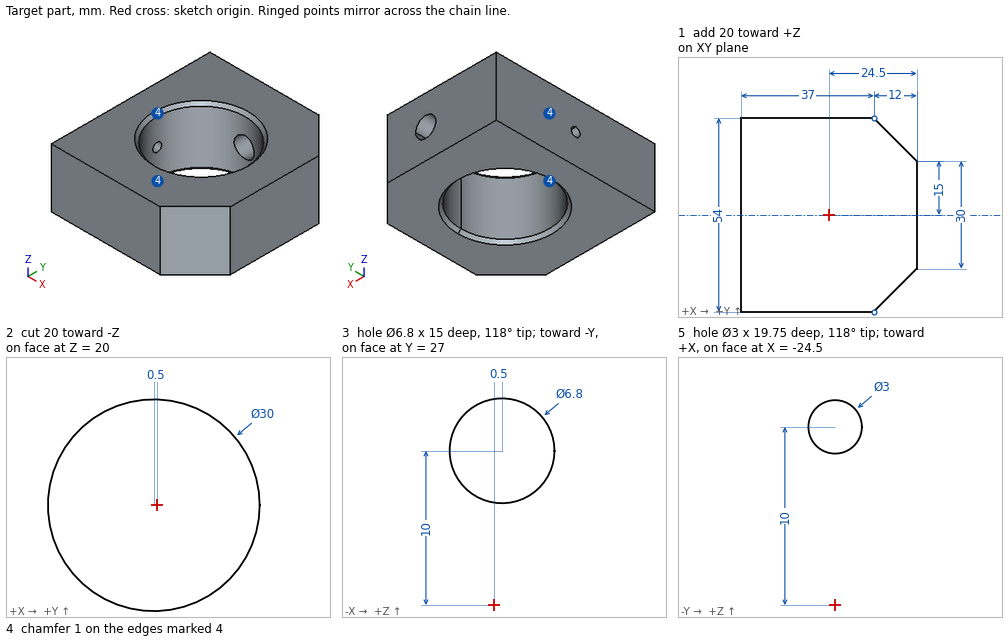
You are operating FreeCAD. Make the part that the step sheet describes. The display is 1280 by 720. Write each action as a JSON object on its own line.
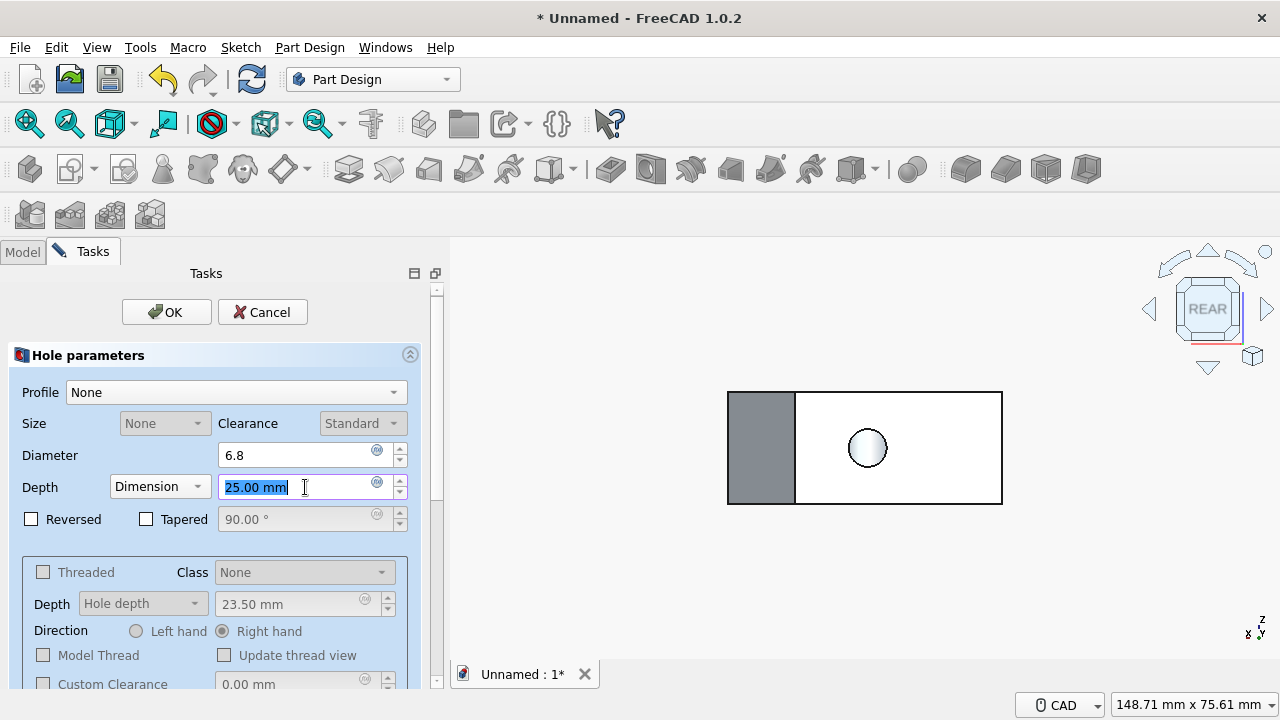
{"action": "type", "text": "15"}
{"action": "key", "text": "Tab"}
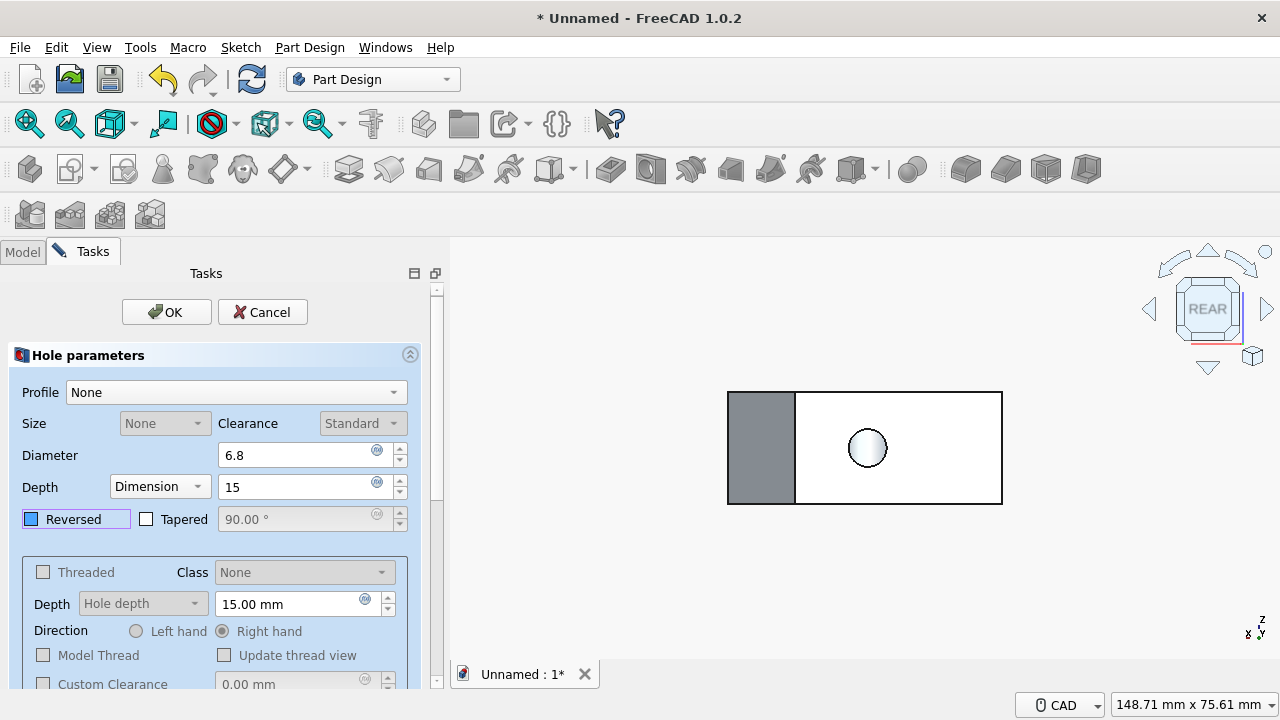
{"action": "left_click", "coordinate": [167, 312]}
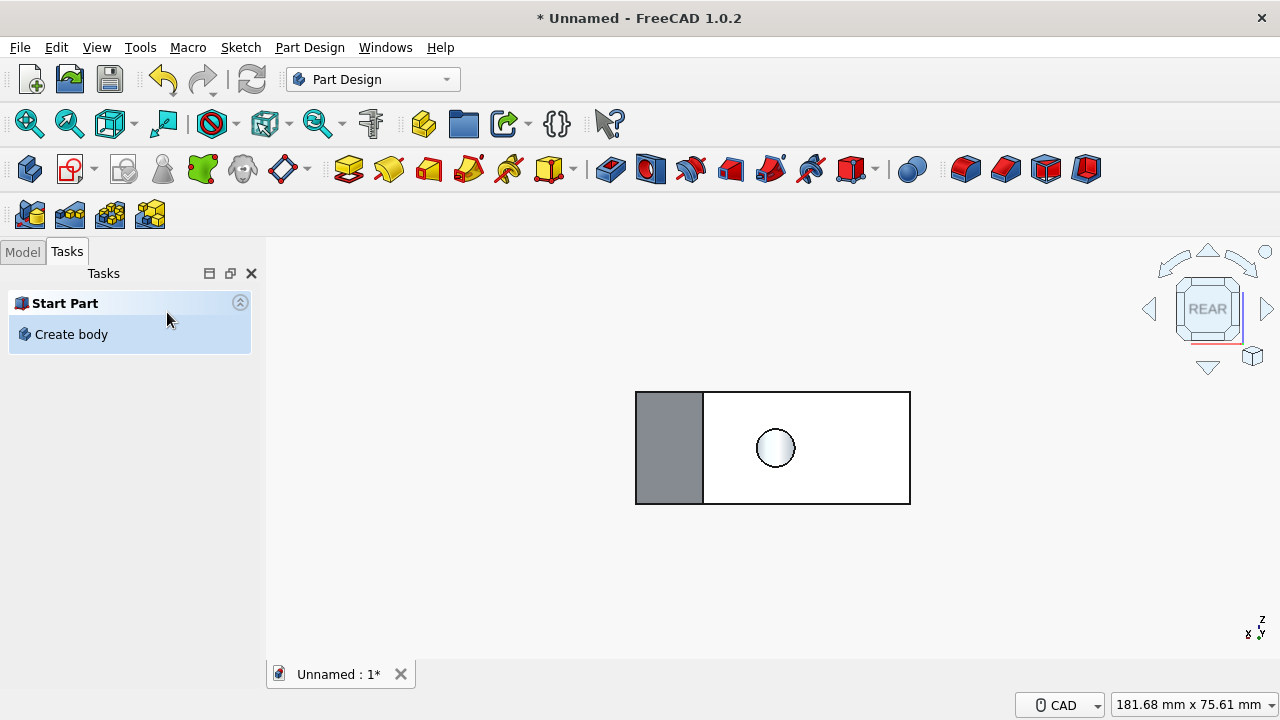
{"action": "left_click", "coordinate": [30, 124]}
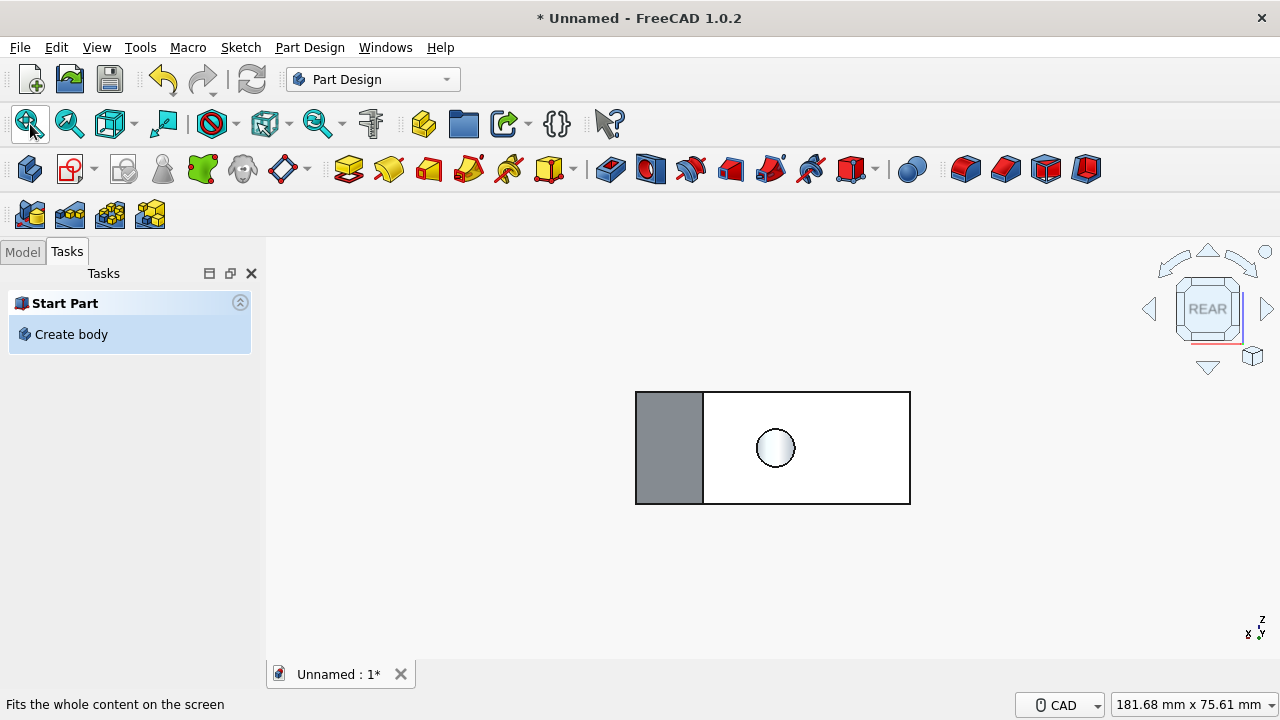
{"action": "key", "text": "0"}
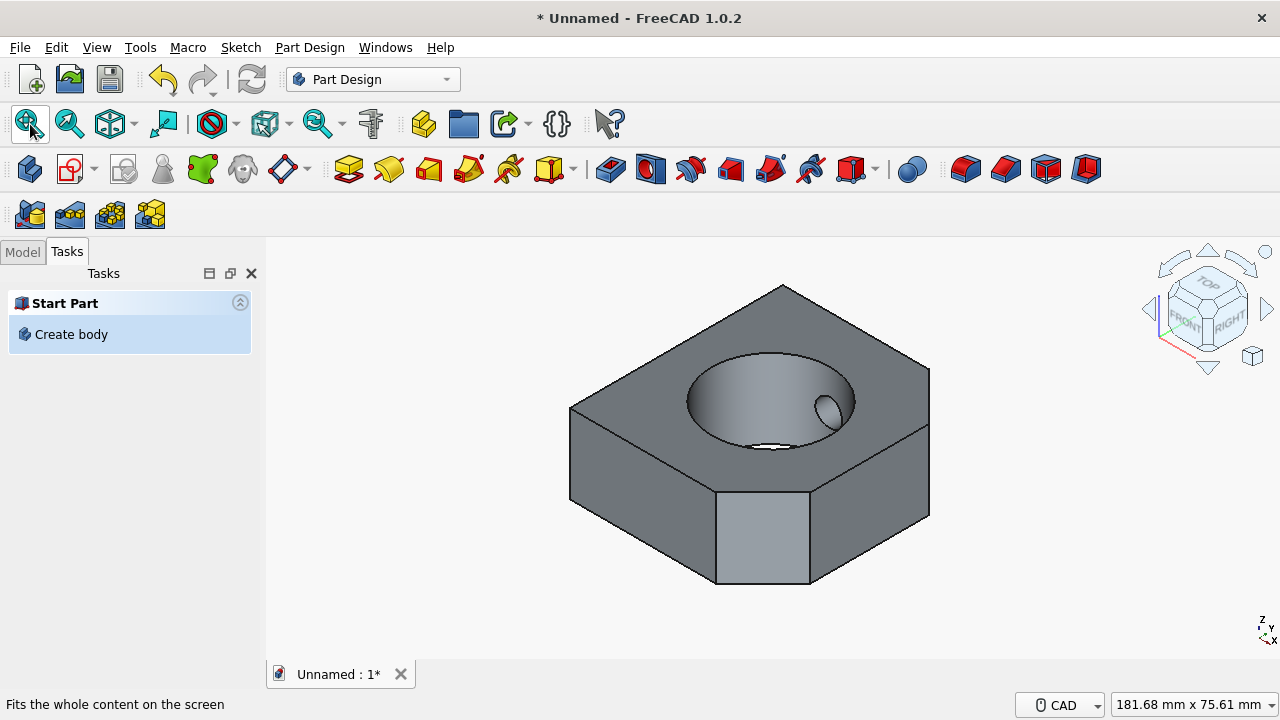
{"action": "left_click", "coordinate": [712, 366]}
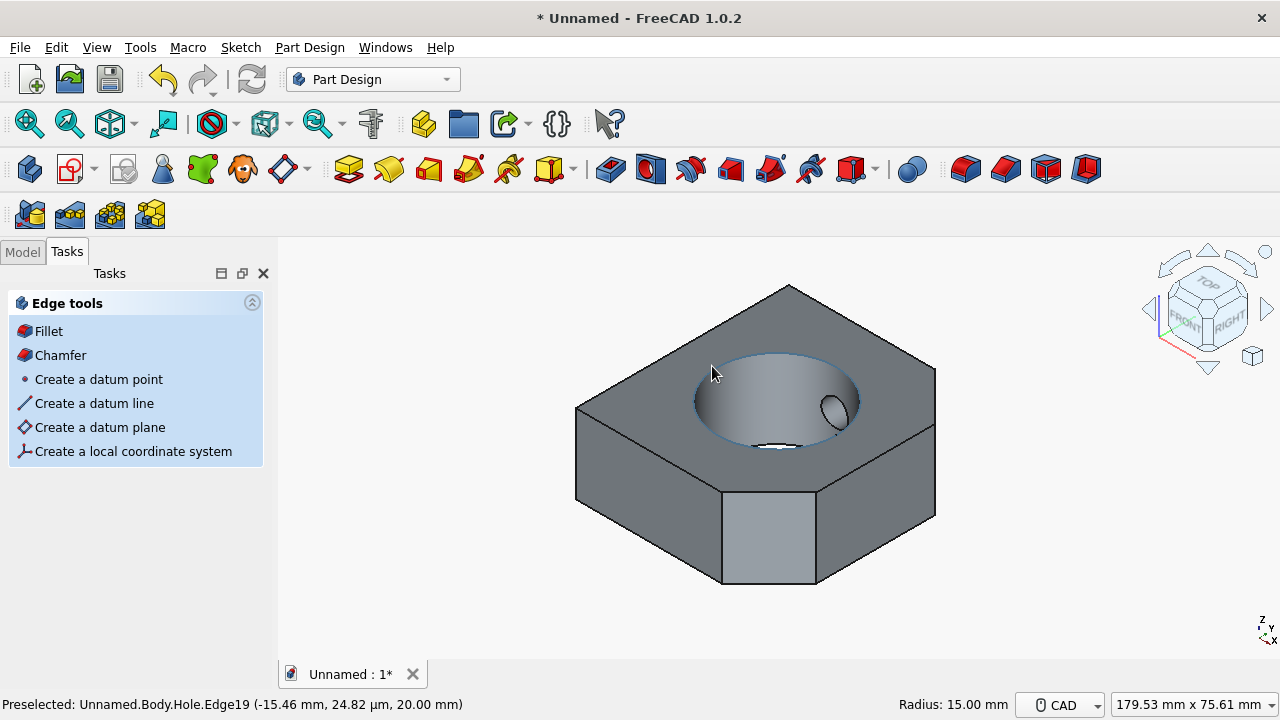
{"action": "key", "text": "2"}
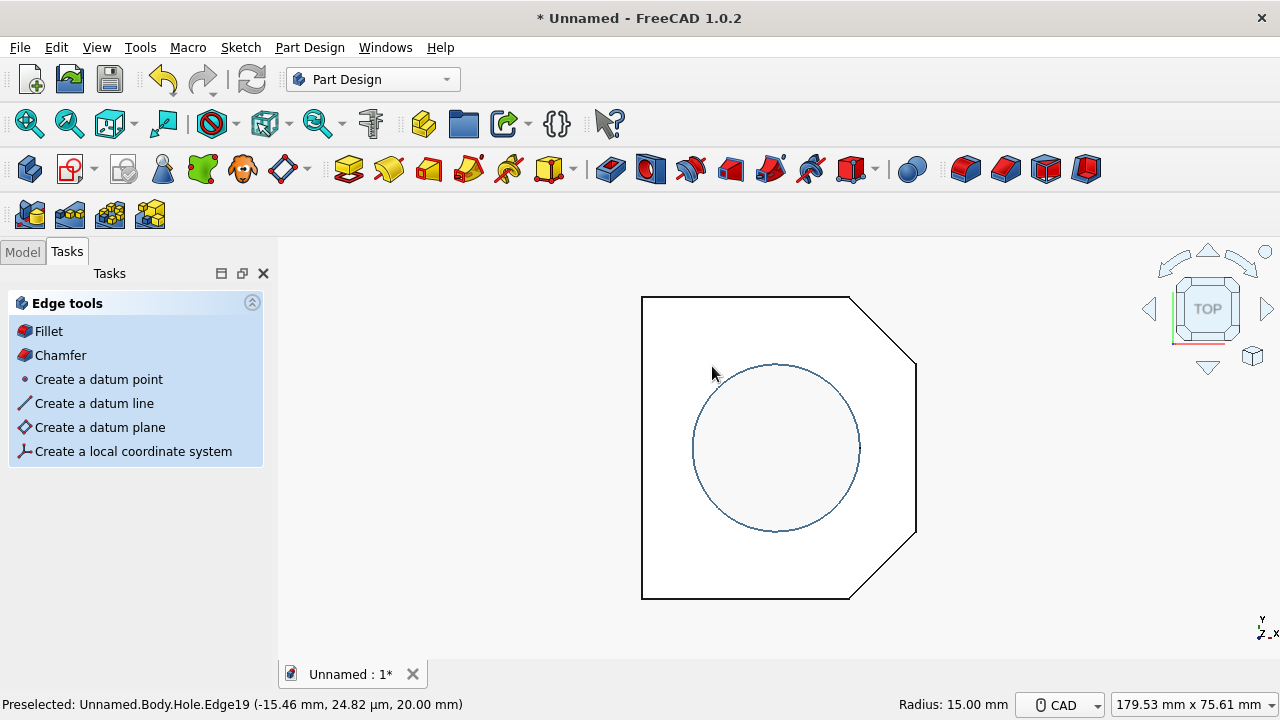
{"action": "key", "text": "1"}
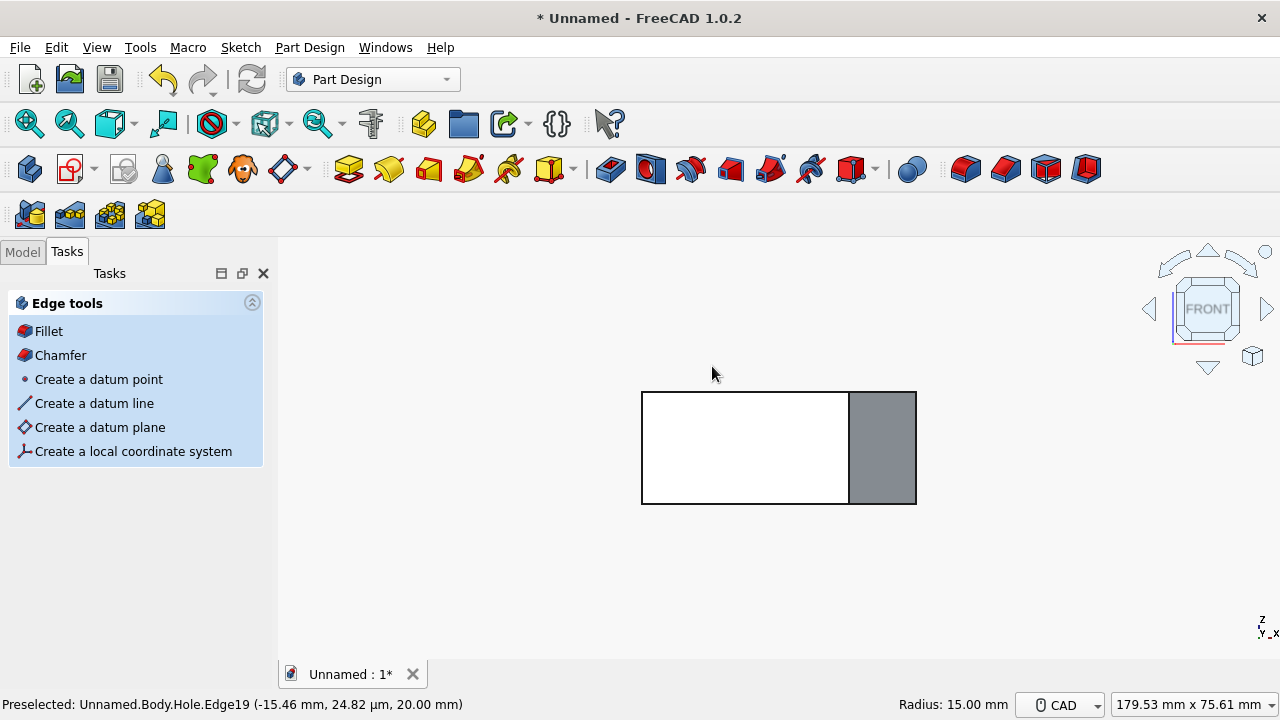
{"action": "key", "text": "v f"}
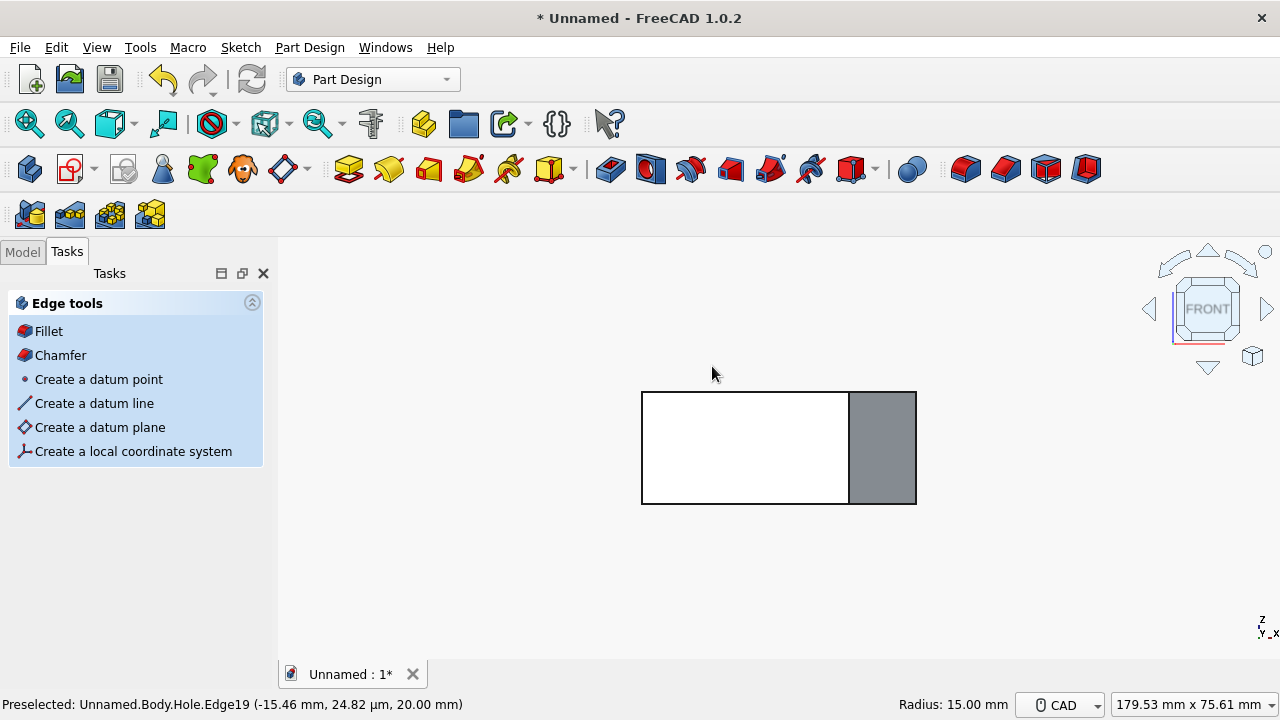
{"action": "key", "text": "3"}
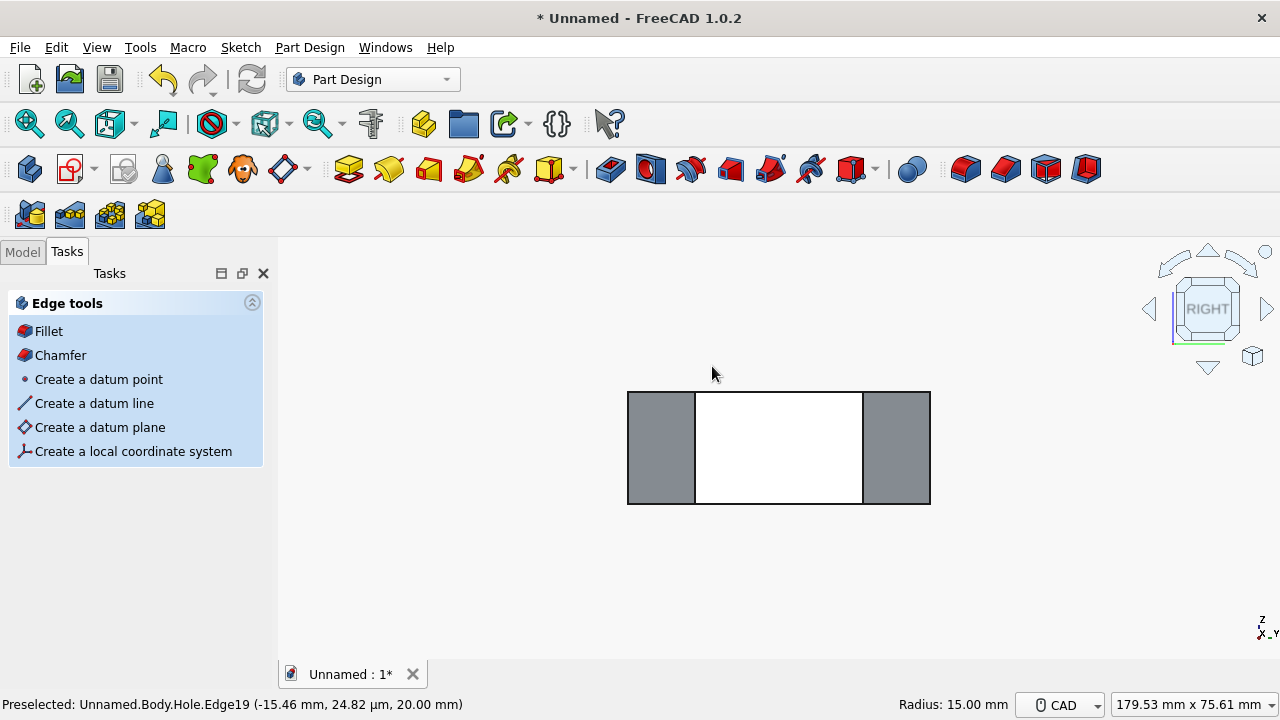
{"action": "key", "text": "v f"}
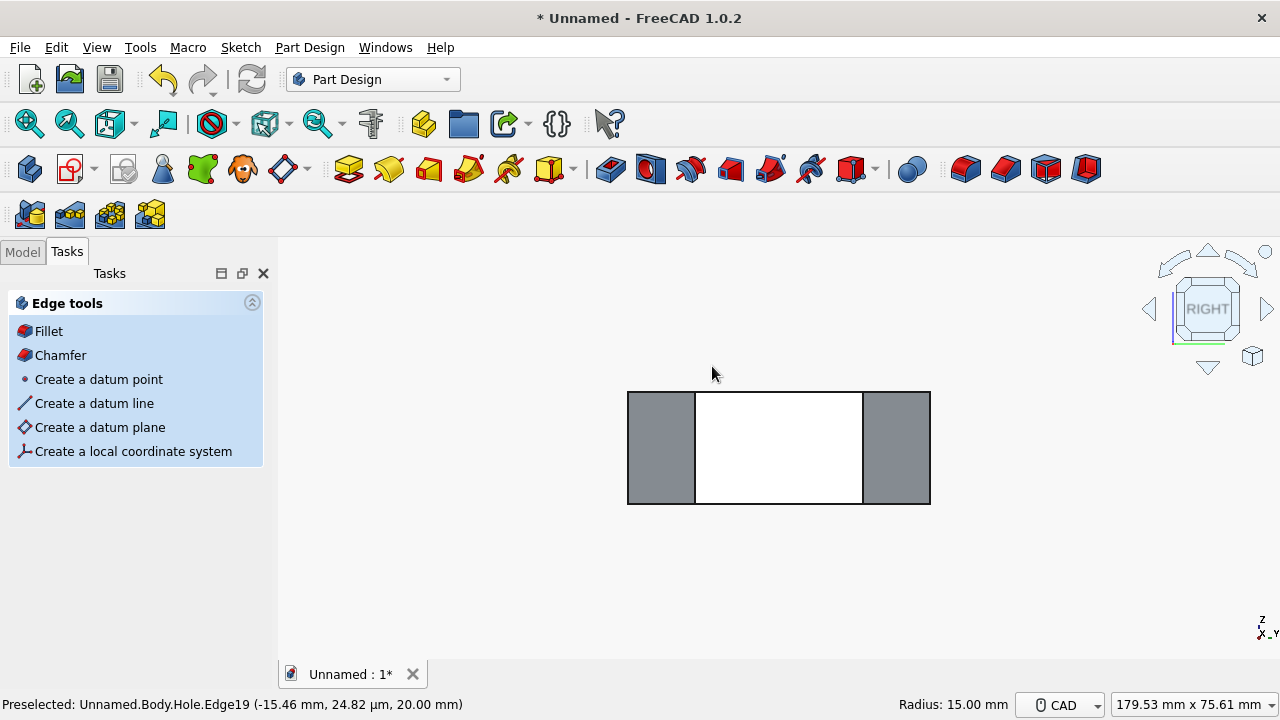
{"action": "key", "text": "5"}